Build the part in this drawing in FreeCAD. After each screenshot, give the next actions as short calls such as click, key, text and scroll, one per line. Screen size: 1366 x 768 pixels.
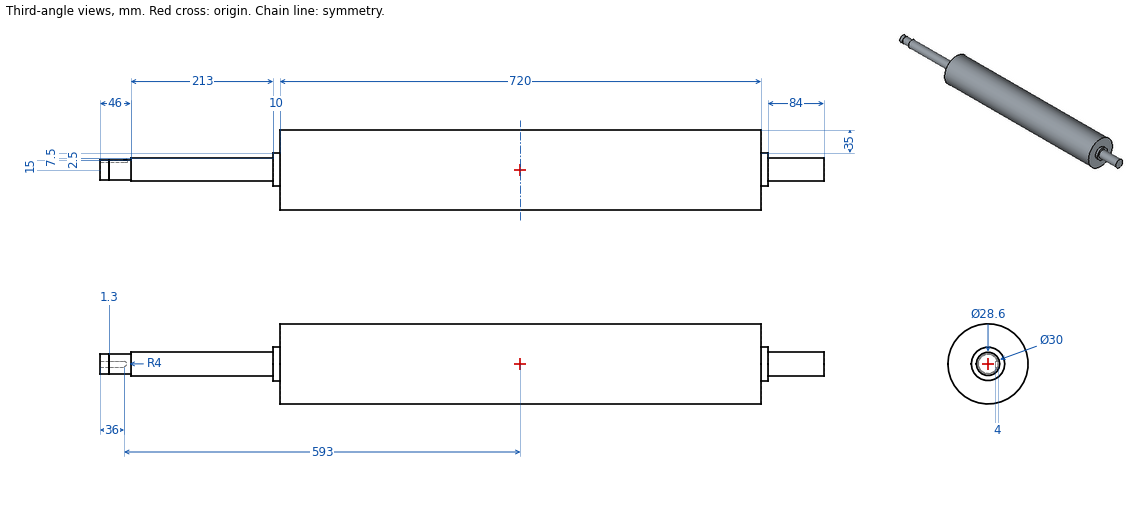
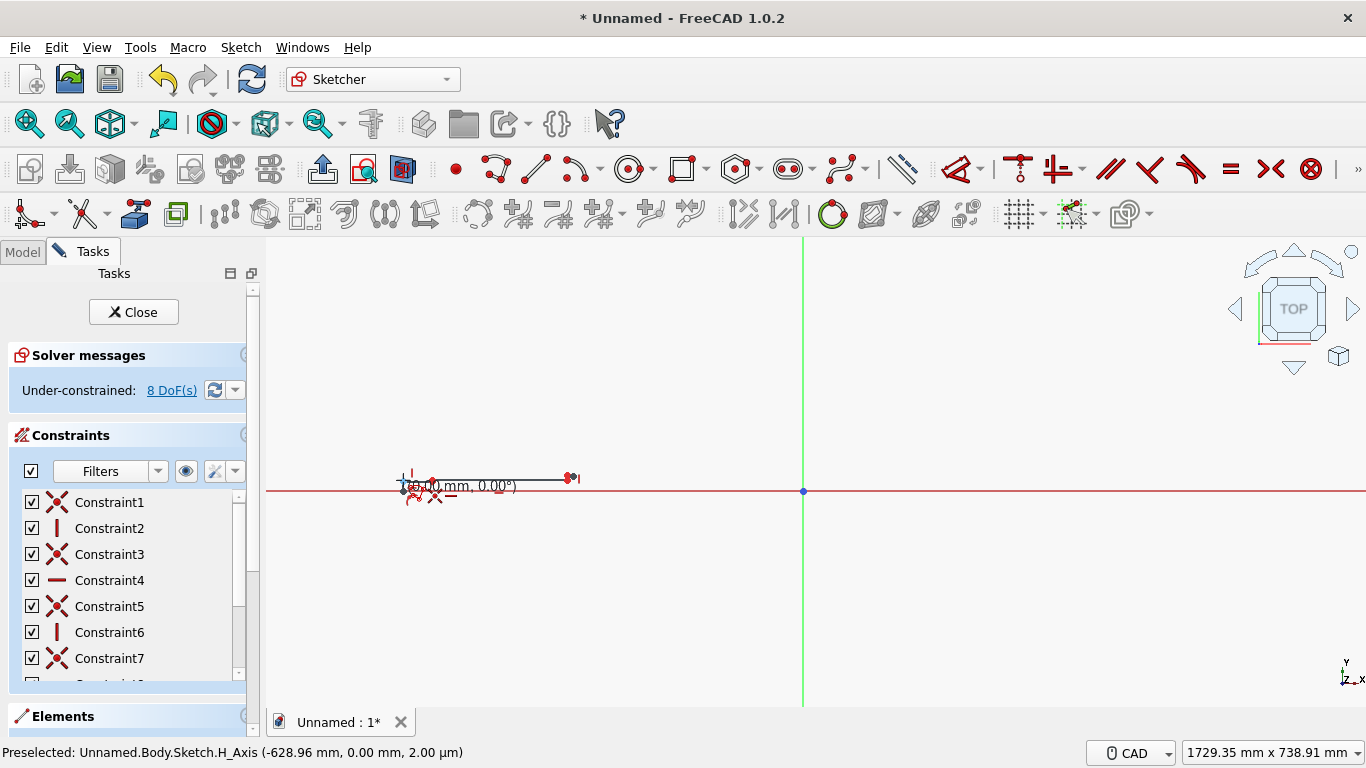
click(1092, 482)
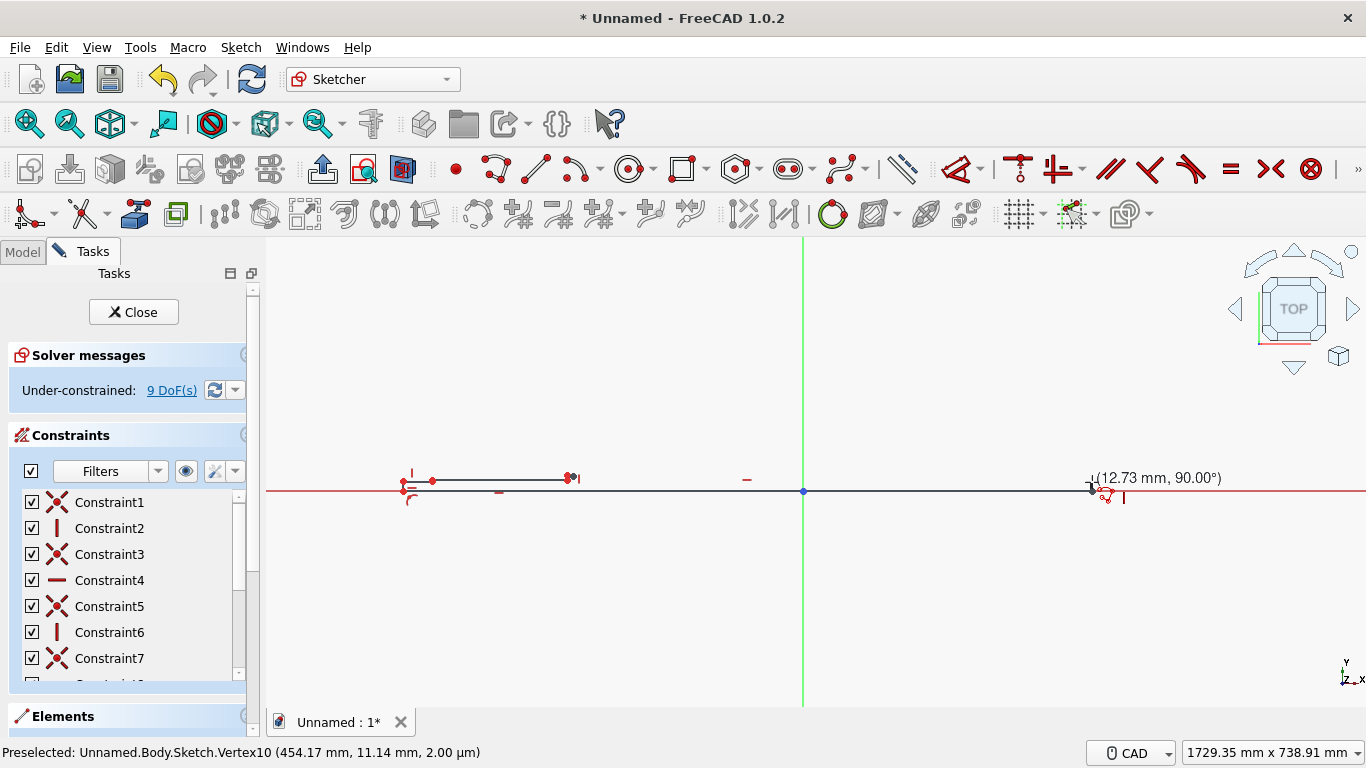
scroll(1092, 480, up, 2)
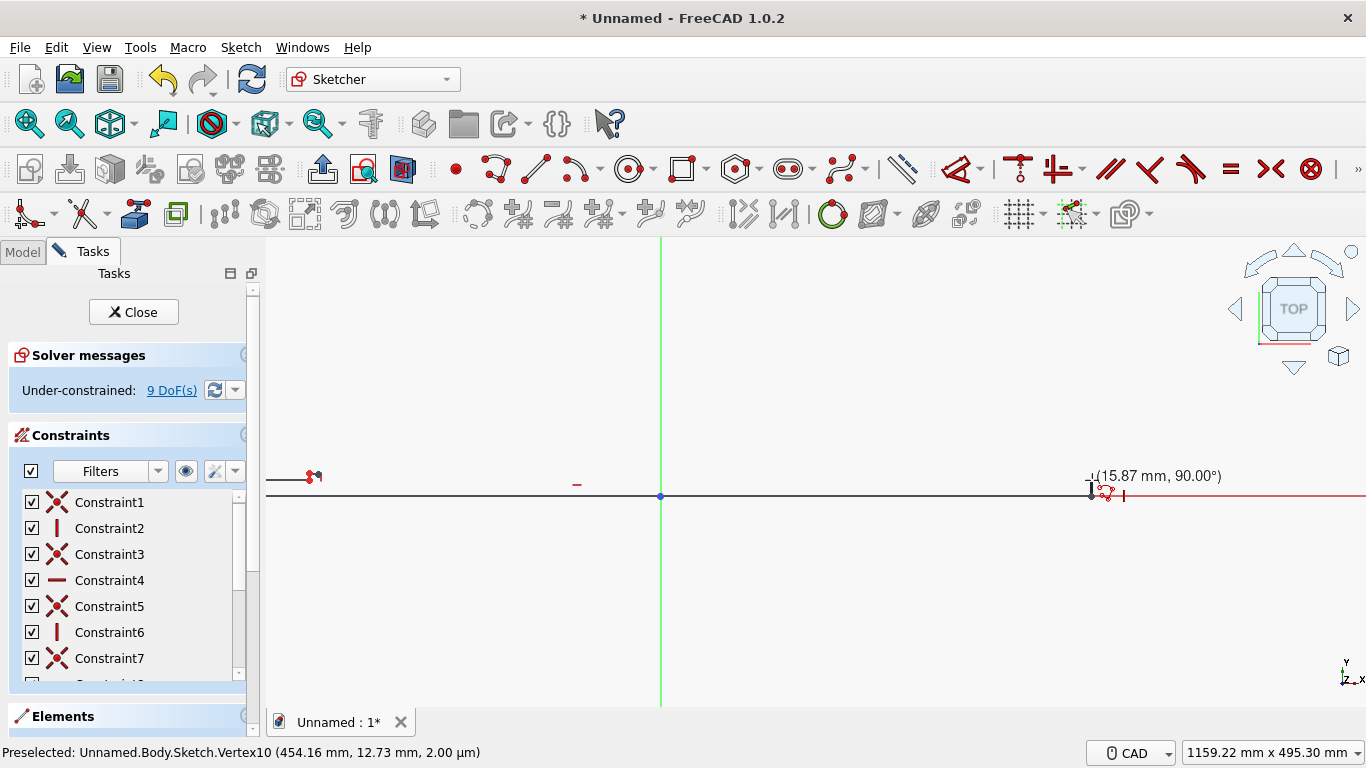
click(1092, 480)
click(1012, 480)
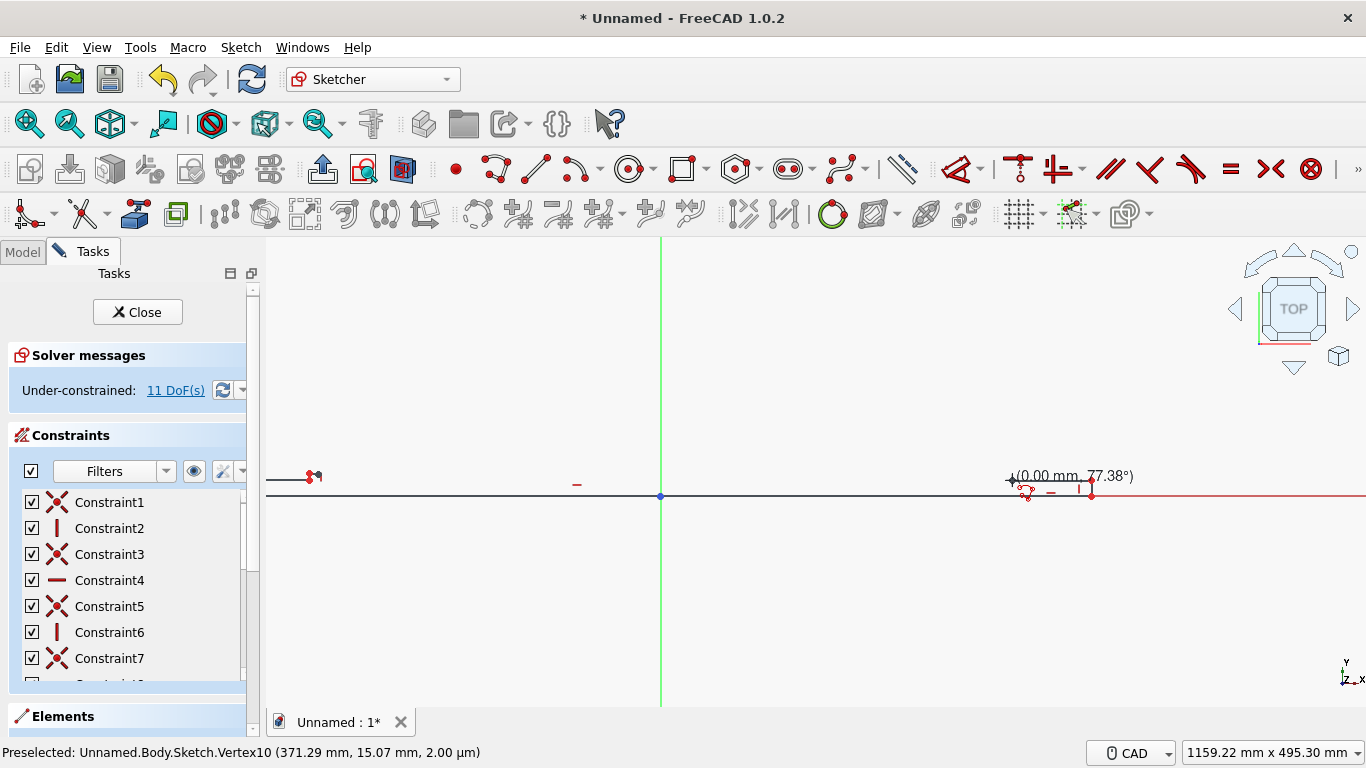
scroll(1012, 473, up, 5)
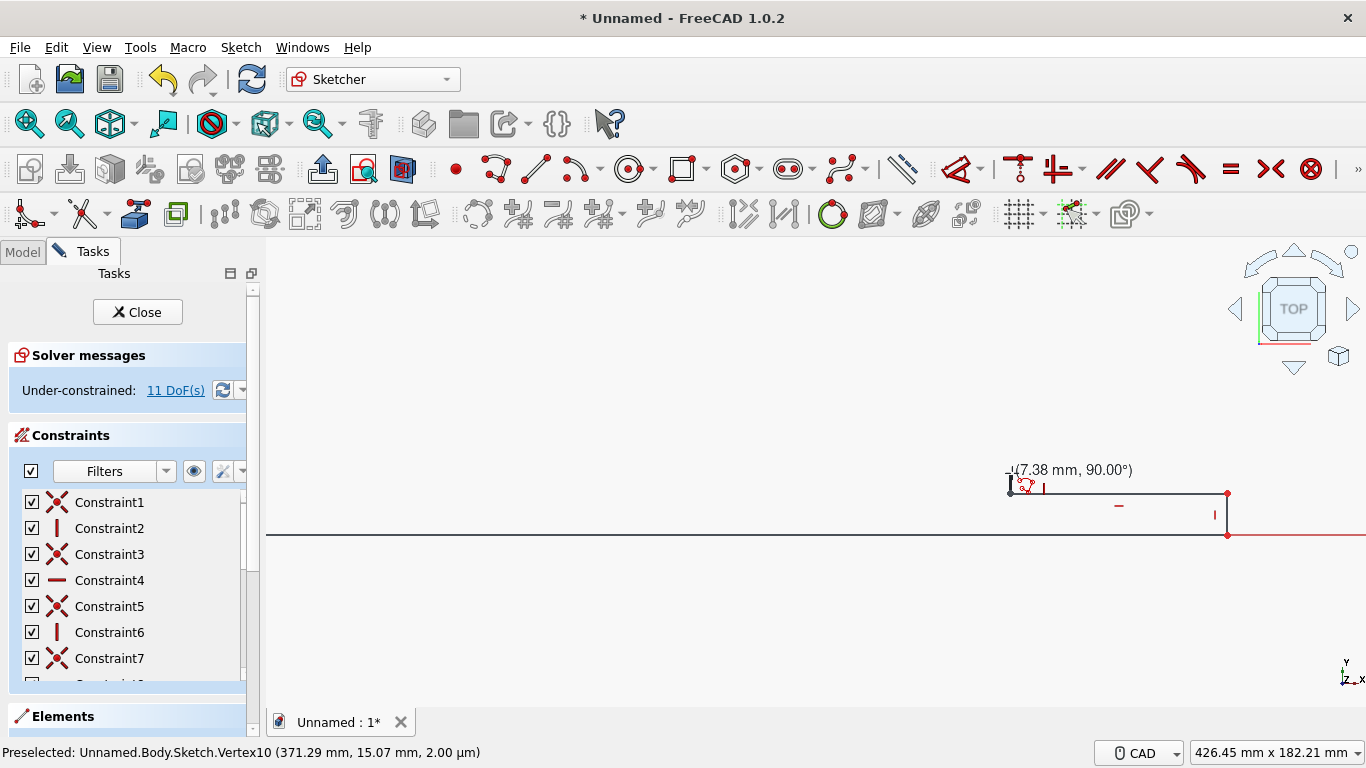
click(1011, 471)
click(984, 471)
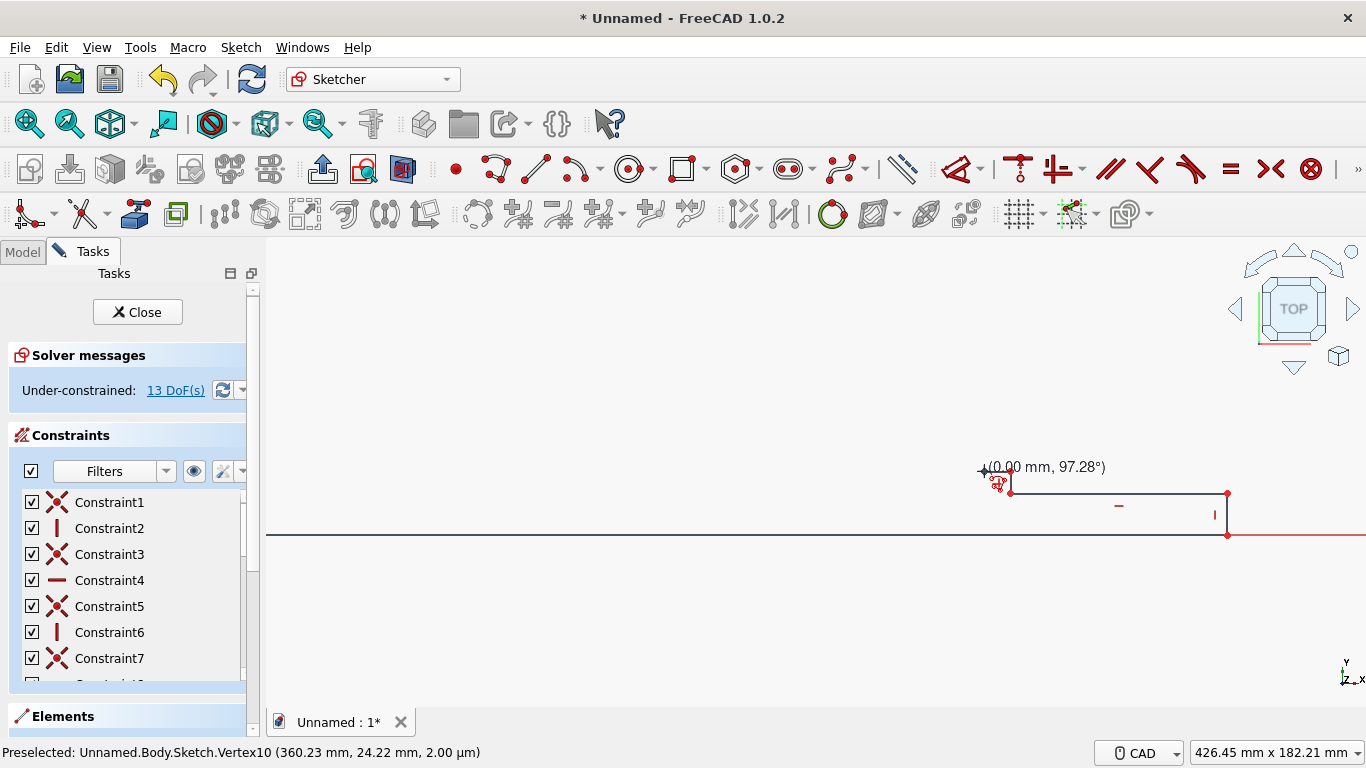
scroll(1048, 477, down, 7)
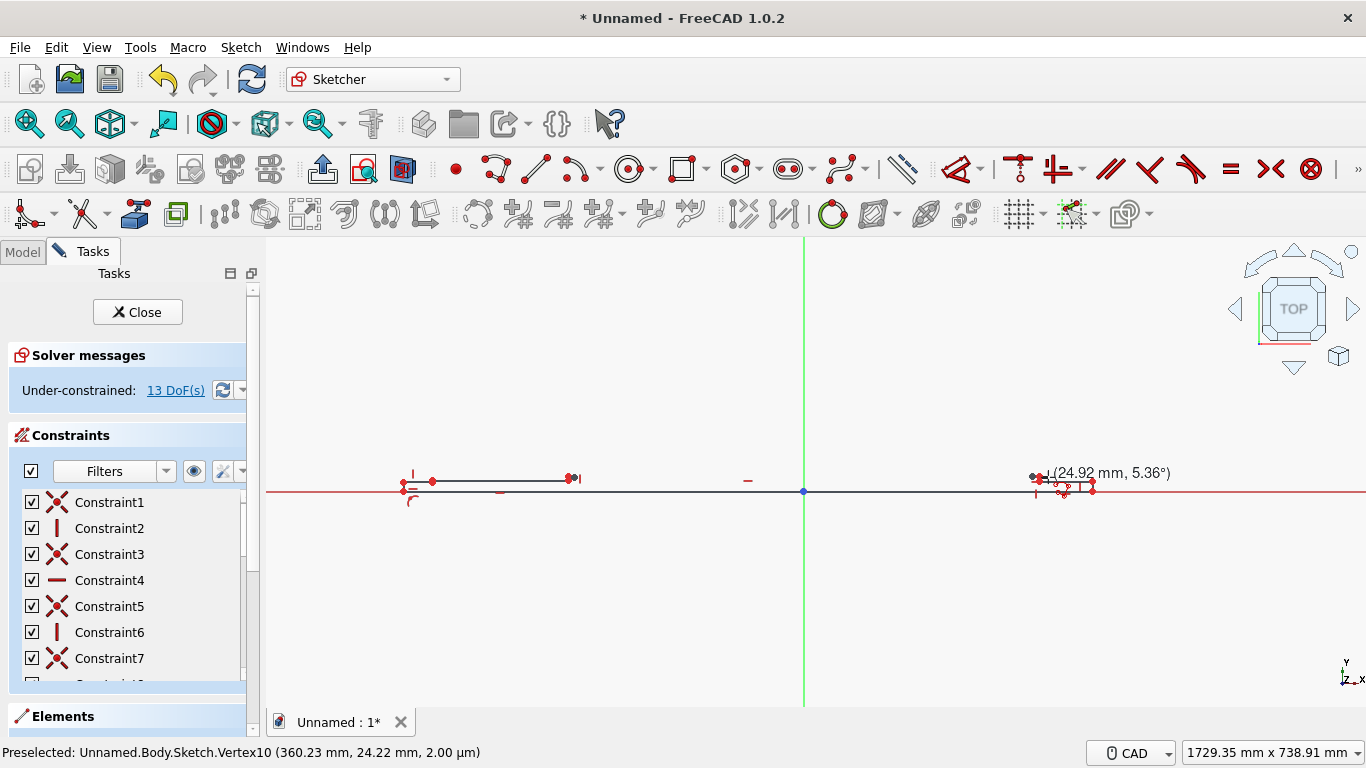
click(1033, 454)
click(575, 454)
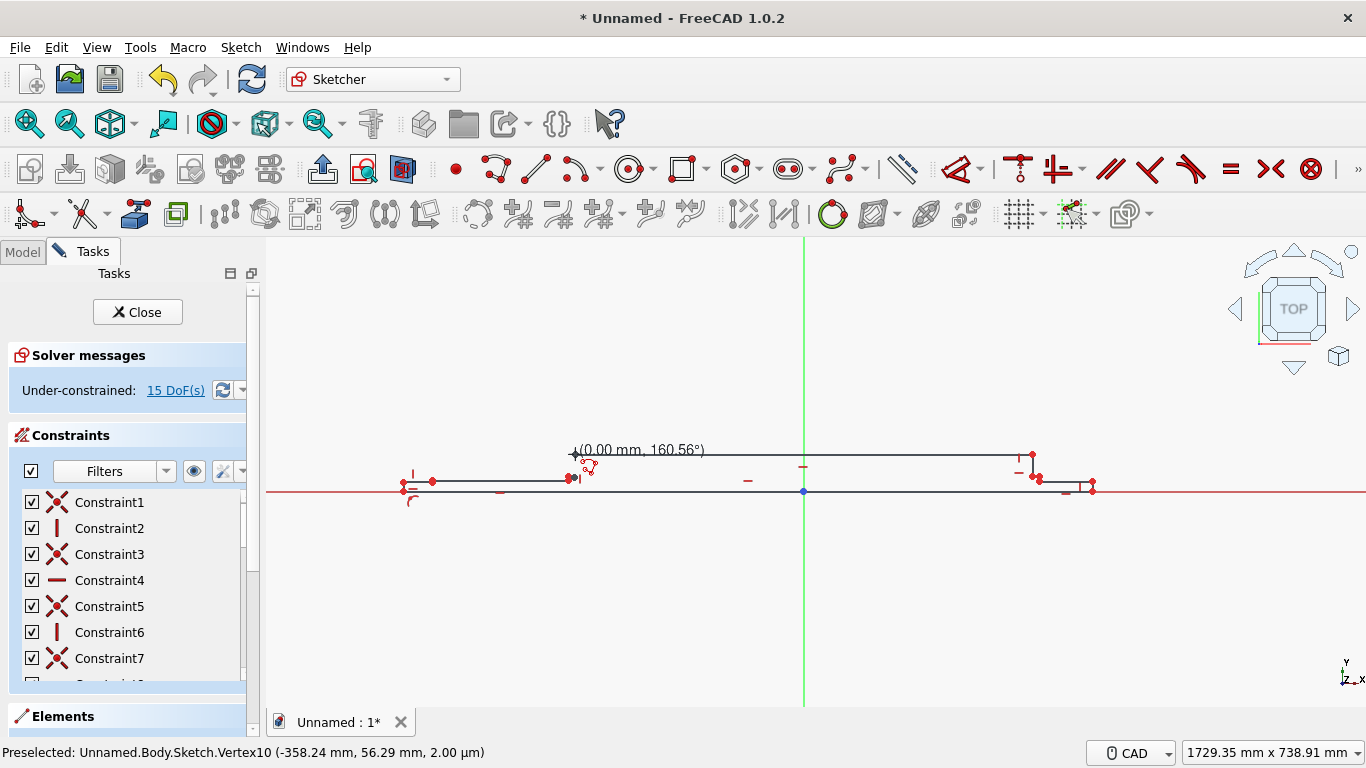
scroll(575, 476, up, 9)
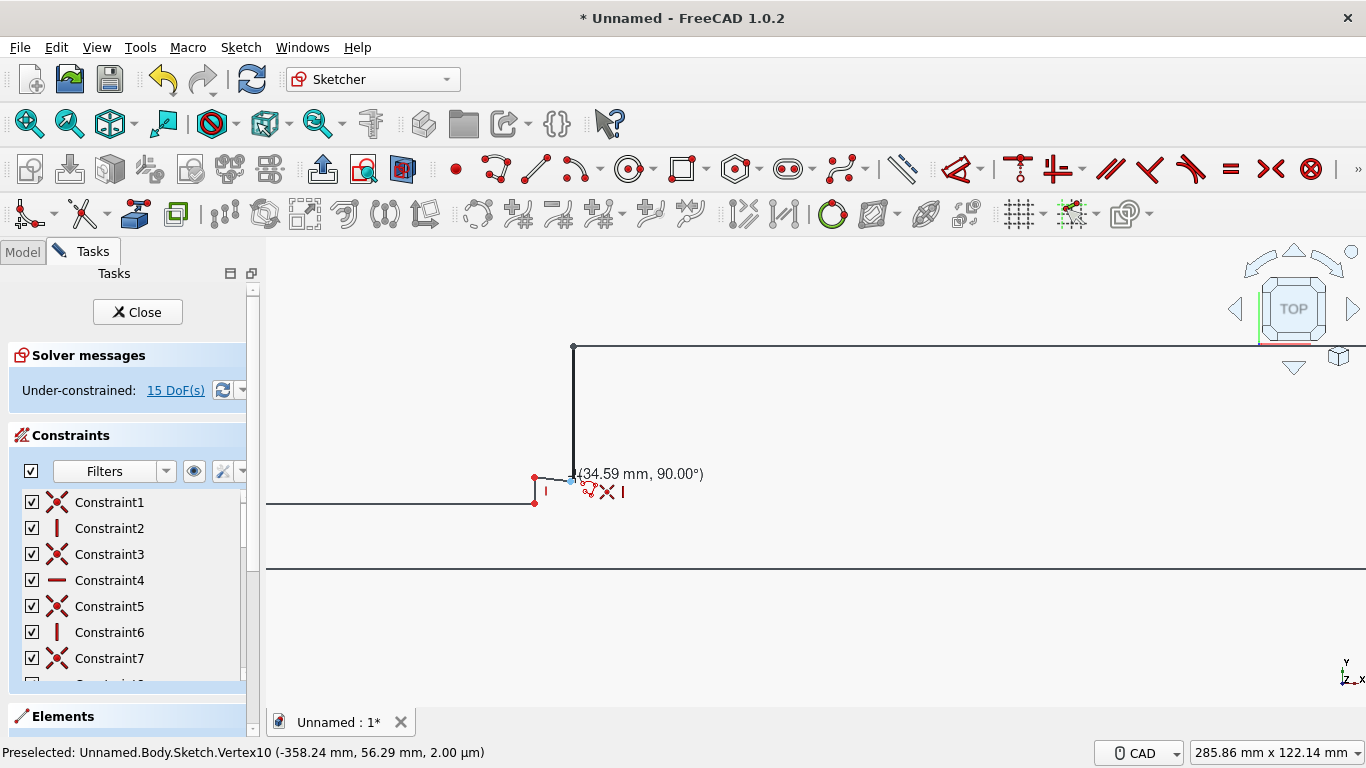
click(570, 481)
key(Escape)
key(Escape)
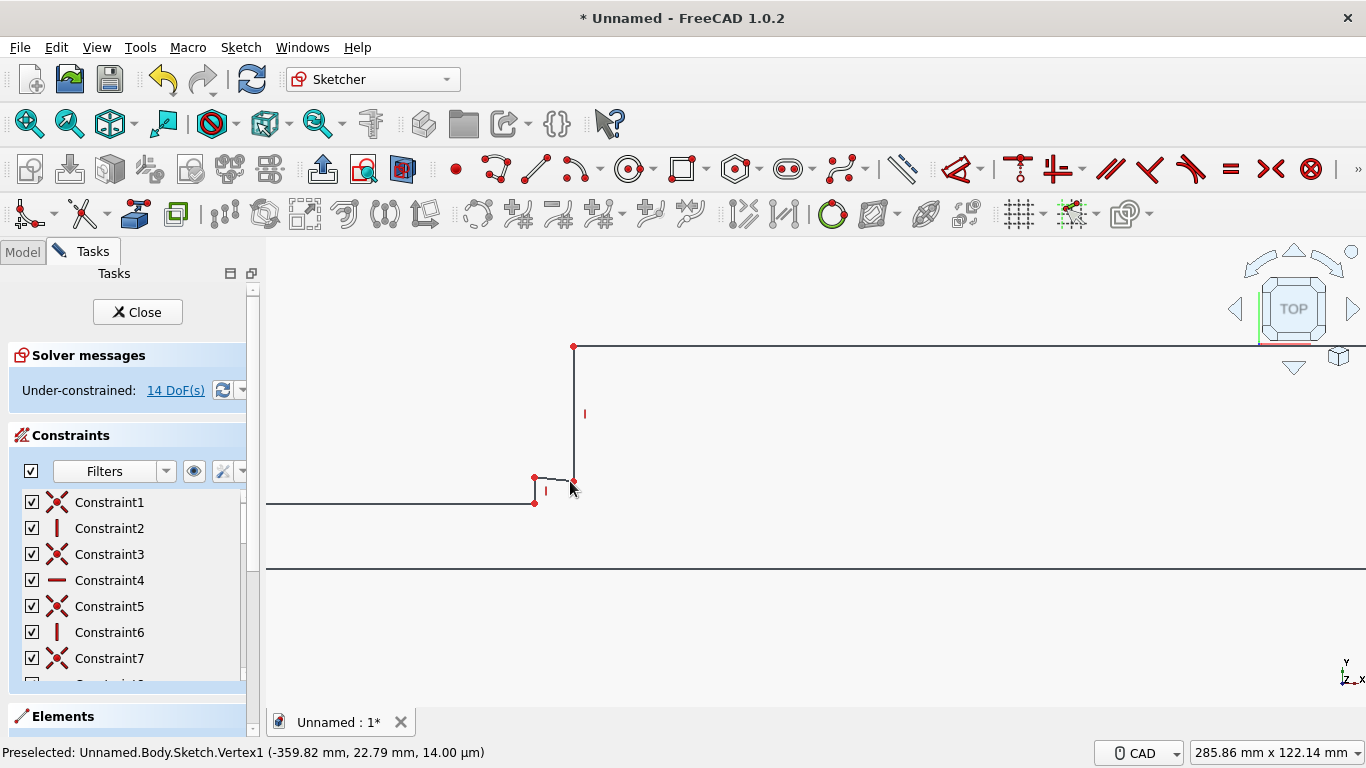
click(562, 480)